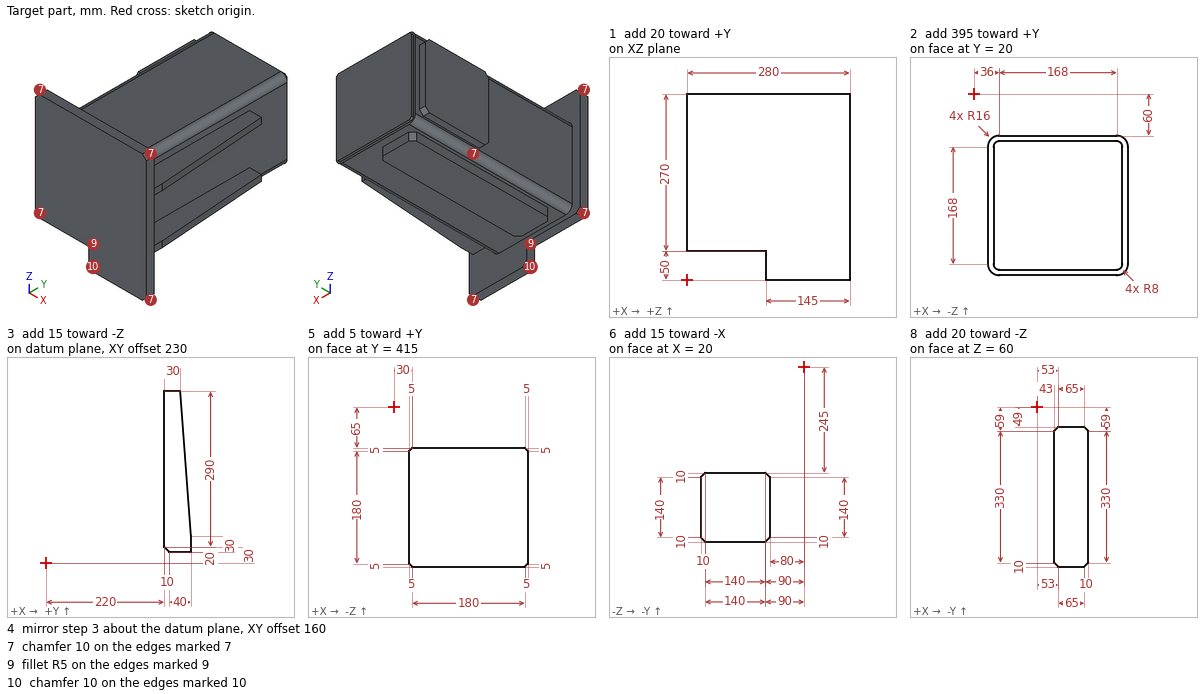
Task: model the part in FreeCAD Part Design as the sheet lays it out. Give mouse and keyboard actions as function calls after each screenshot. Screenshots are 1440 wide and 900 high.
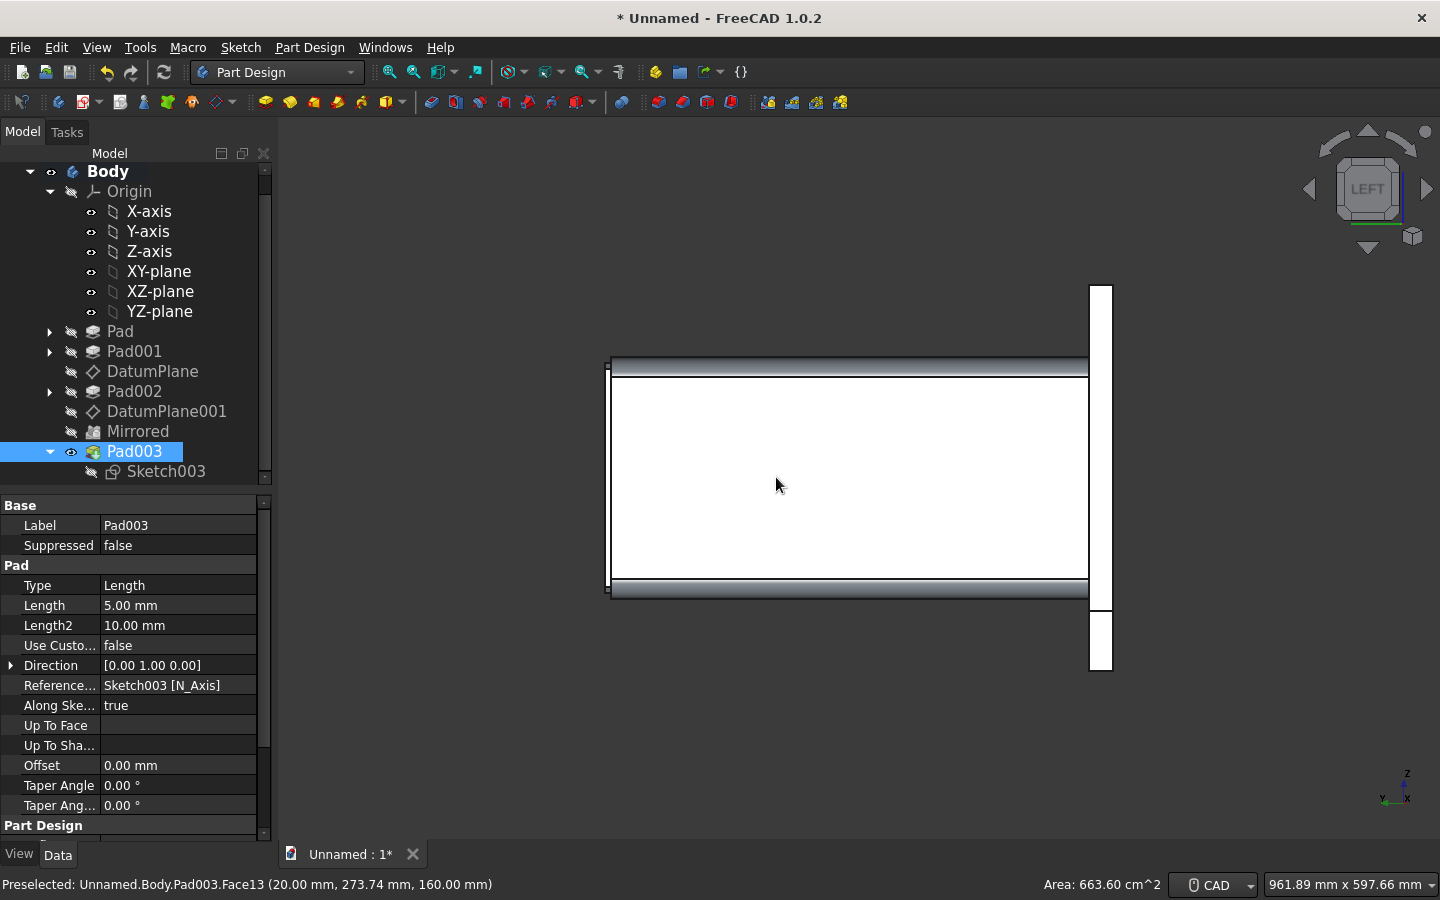
click(84, 102)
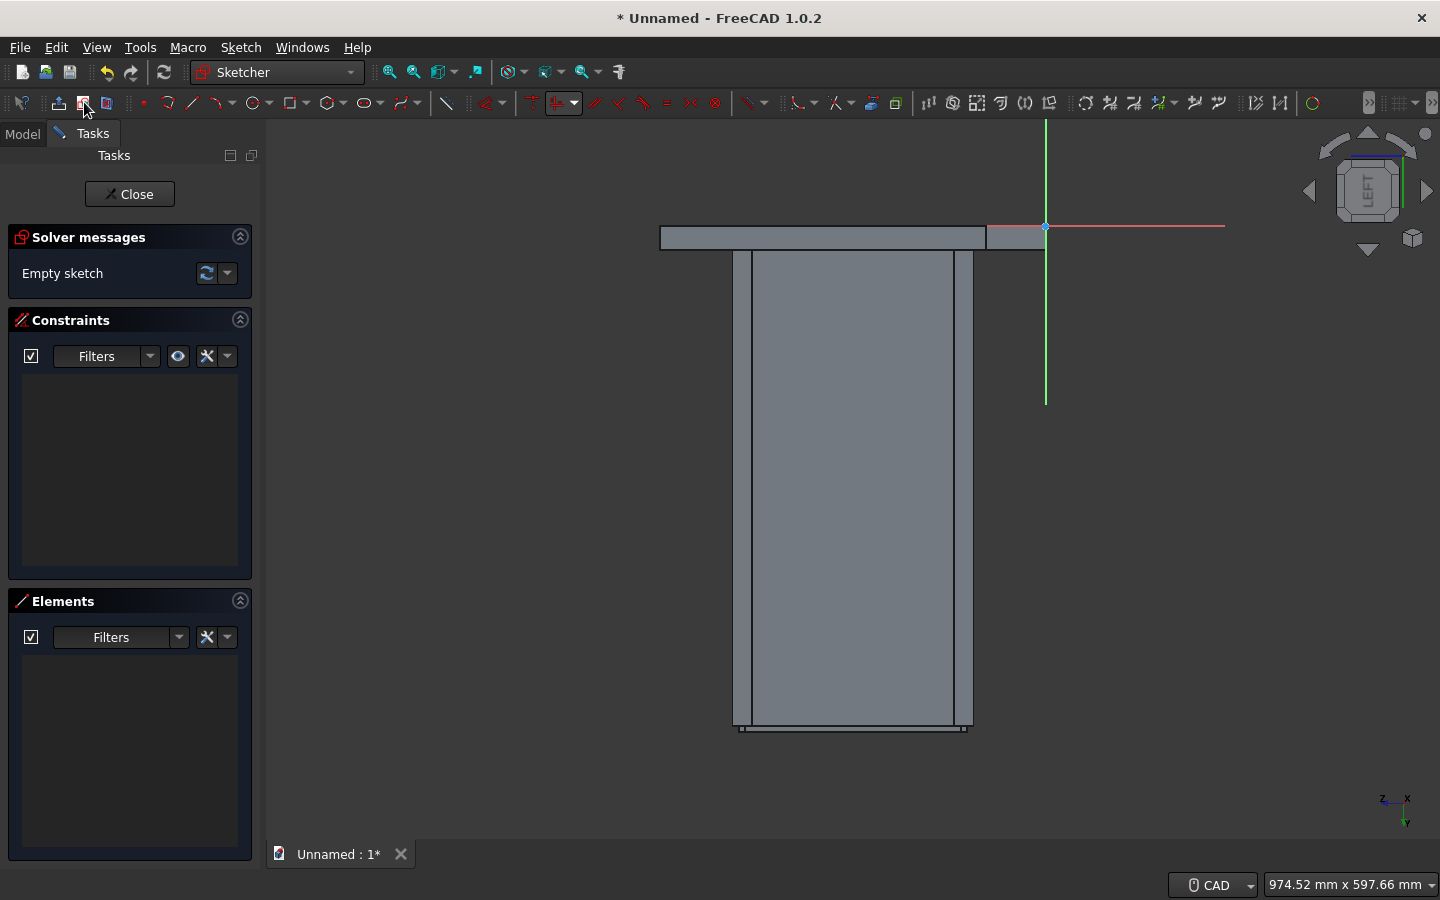
click(108, 104)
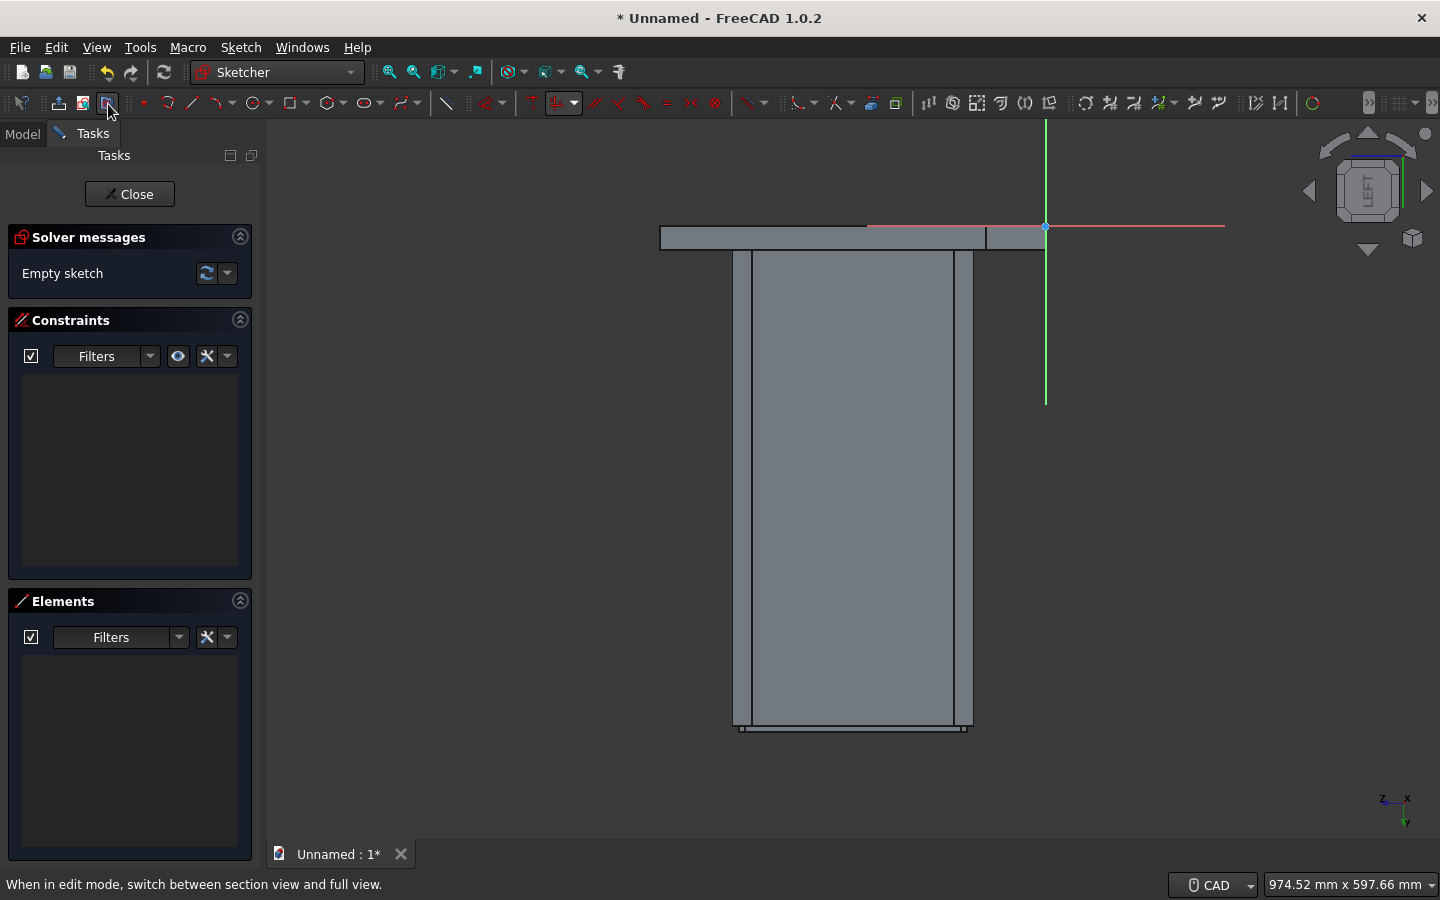
scroll(909, 731, up, 4)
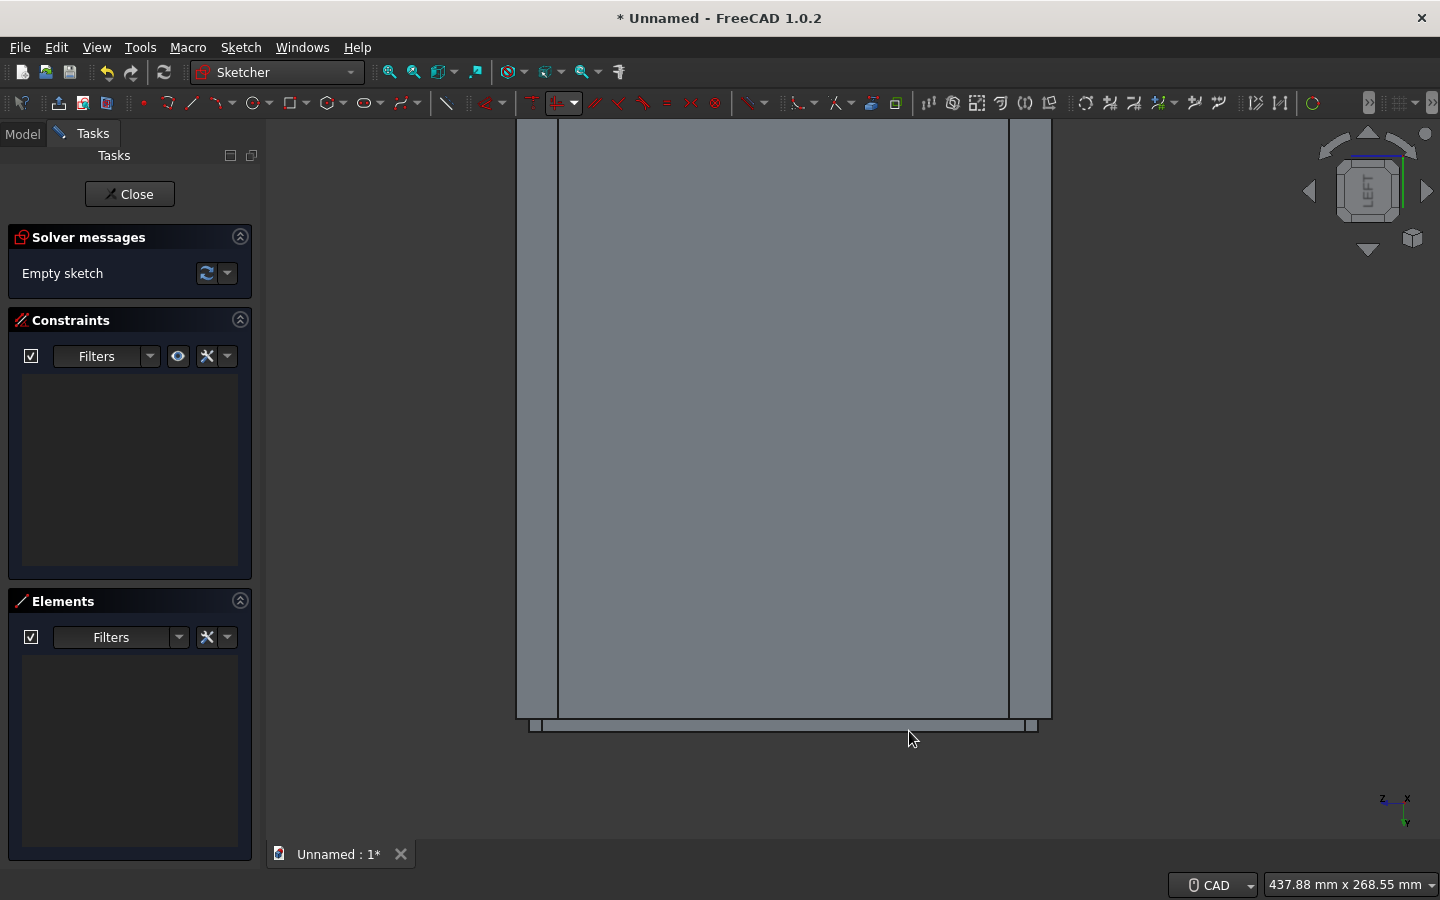
click(168, 104)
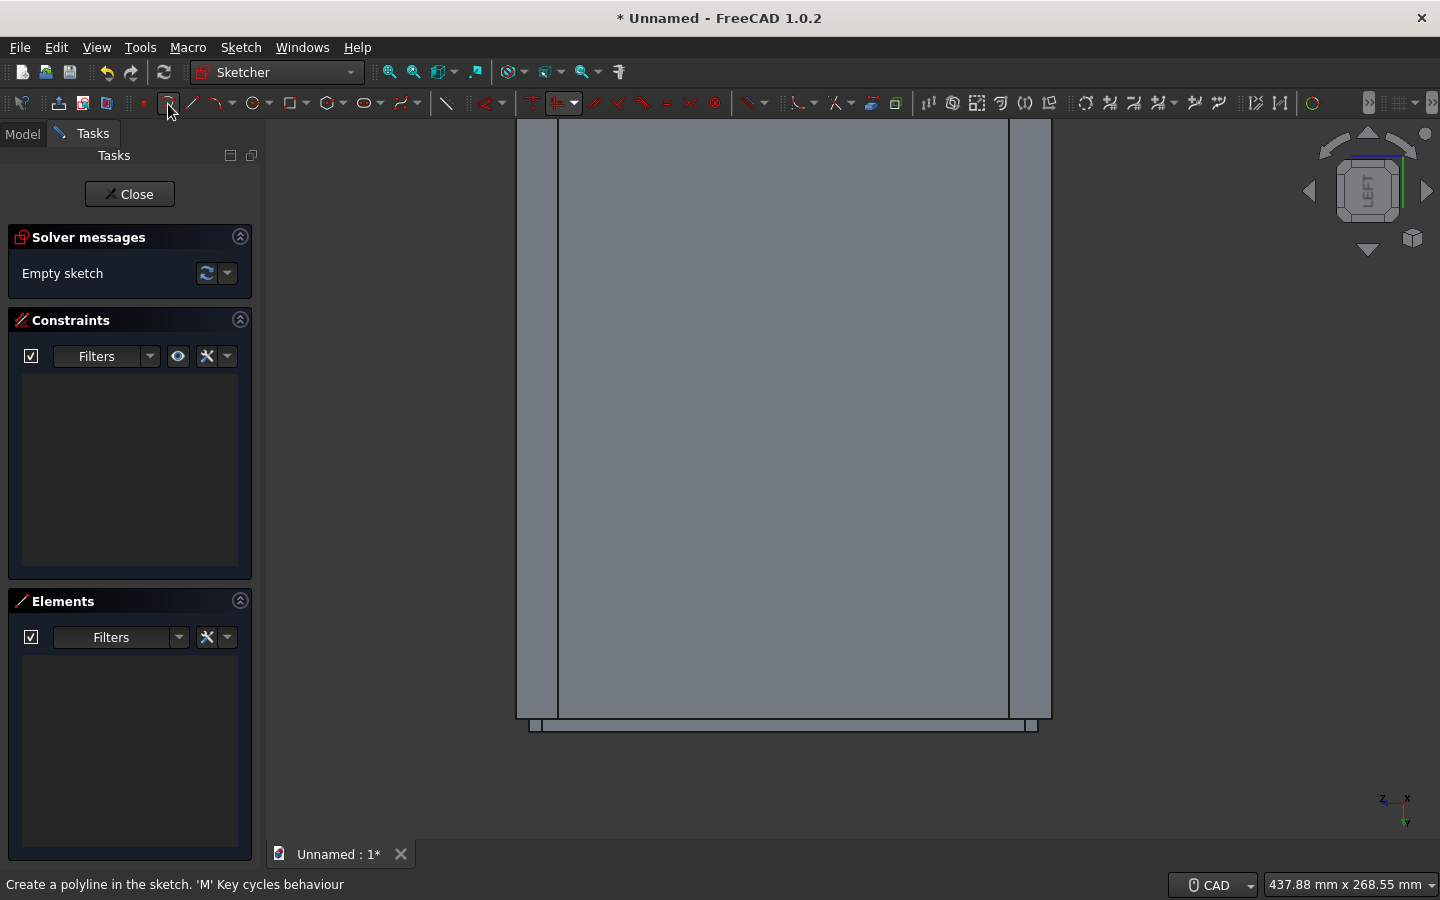
click(971, 263)
click(596, 263)
click(569, 290)
click(569, 665)
click(596, 692)
click(971, 692)
click(998, 665)
click(998, 290)
click(971, 264)
key(Escape)
key(Escape)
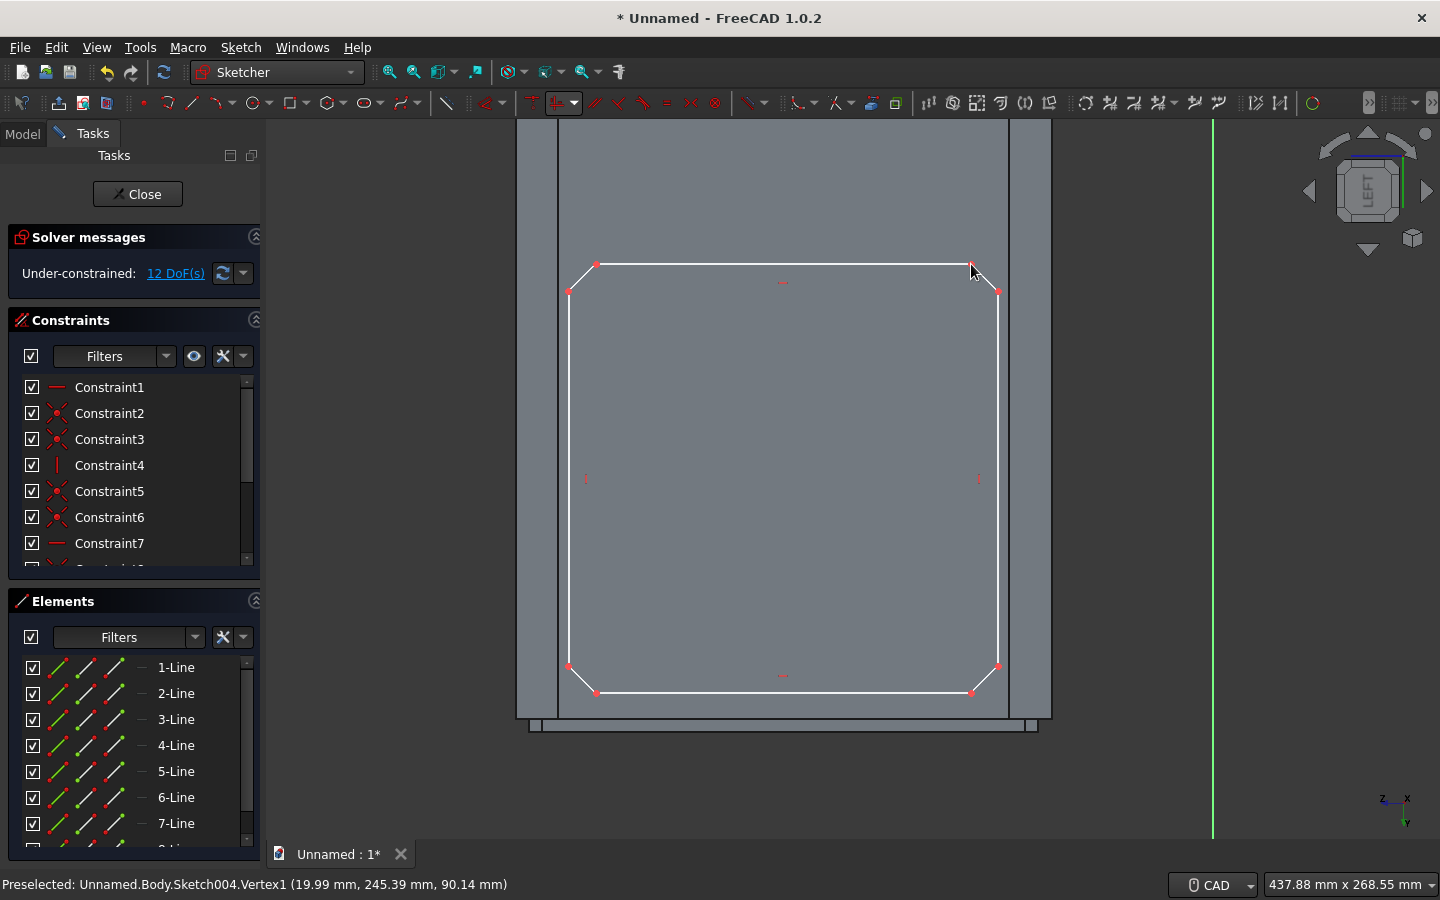
click(486, 104)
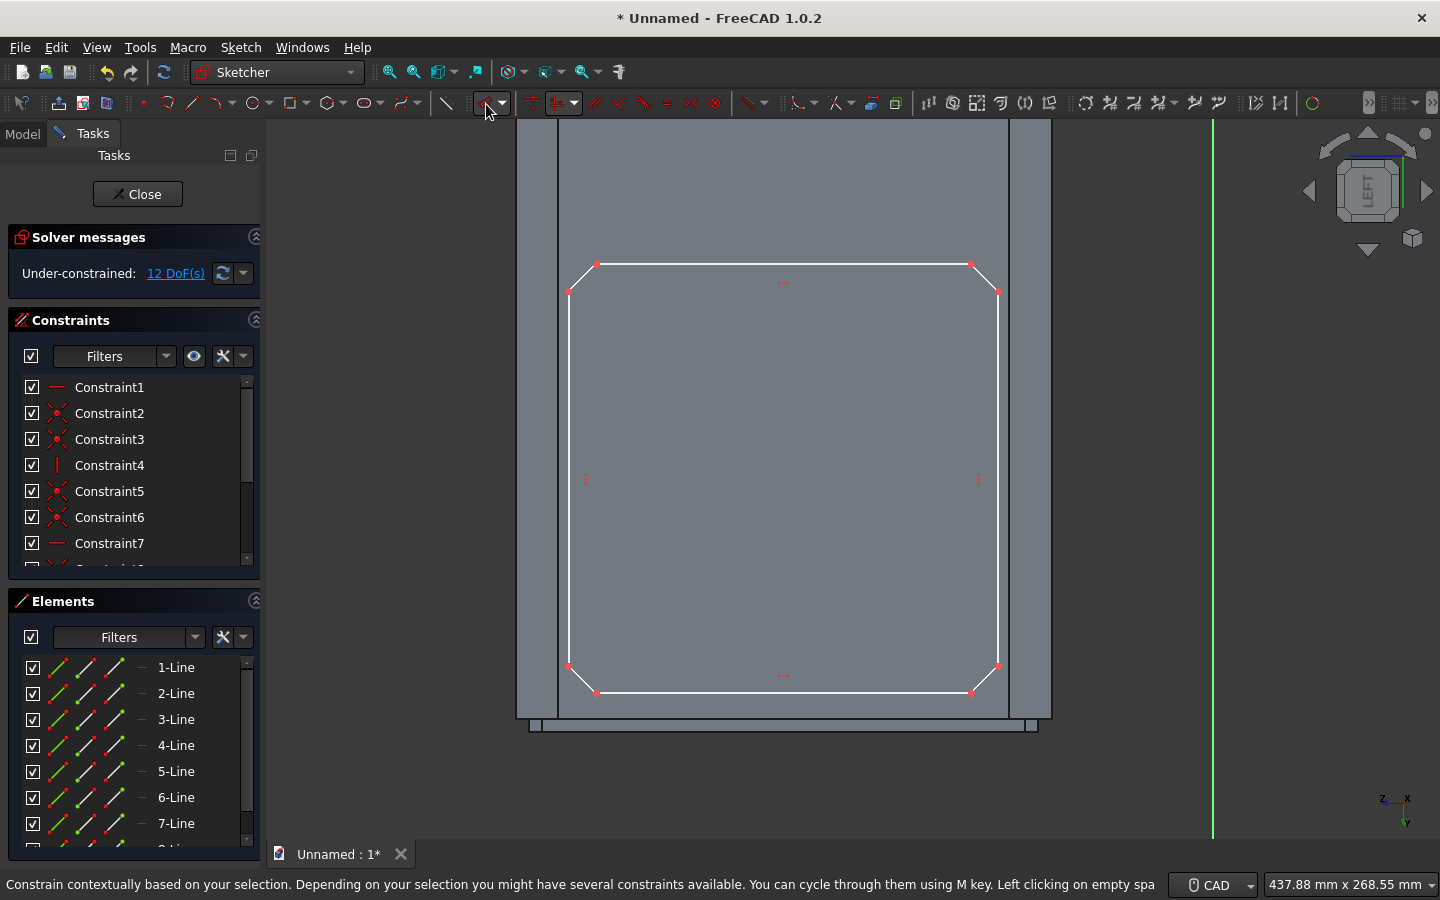
click(858, 264)
click(783, 230)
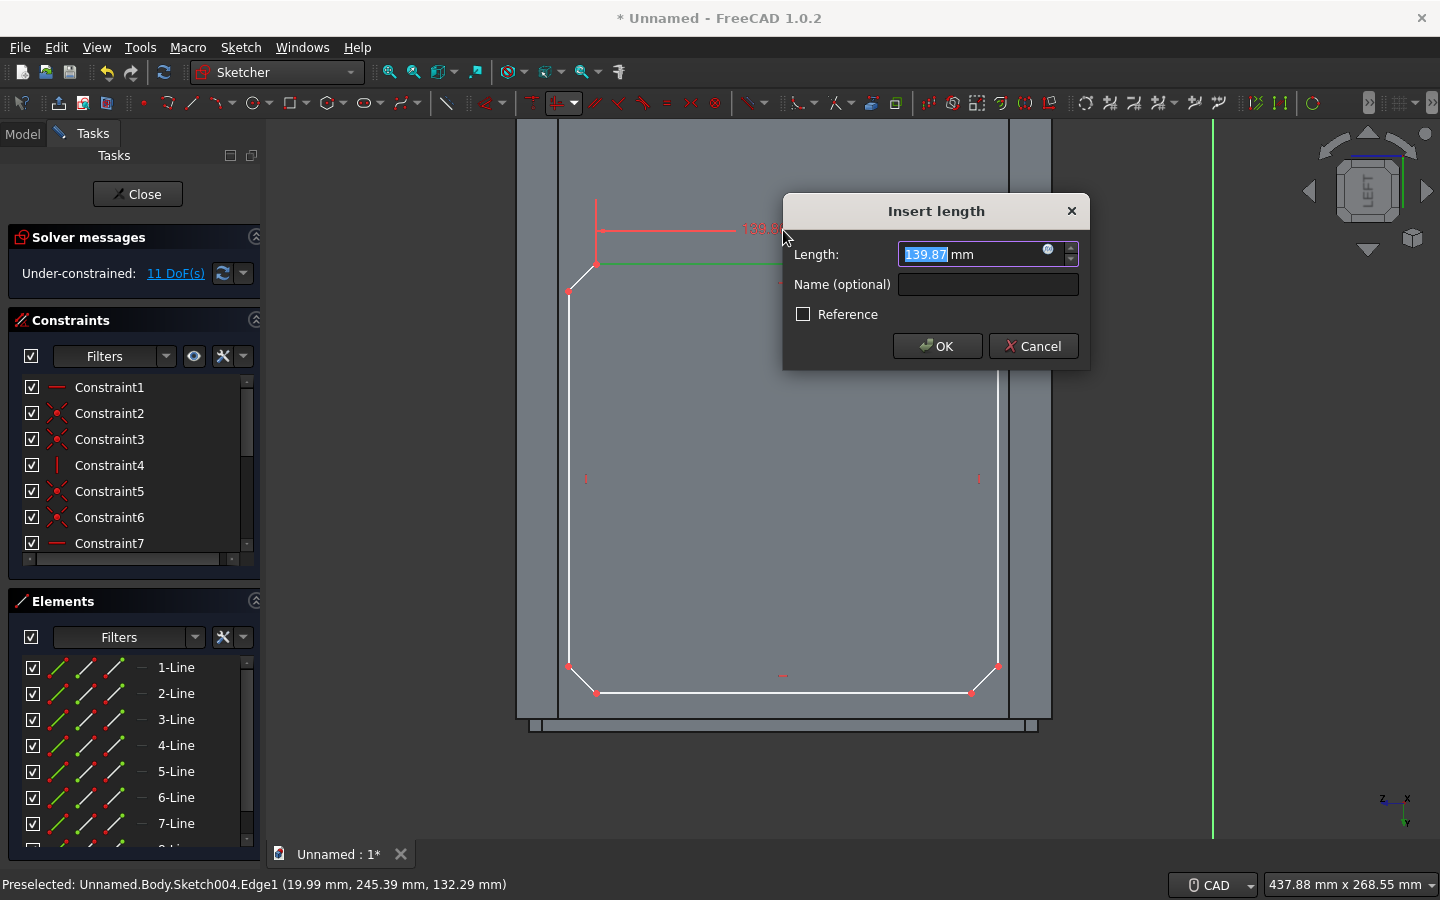
text(140)
key(Return)